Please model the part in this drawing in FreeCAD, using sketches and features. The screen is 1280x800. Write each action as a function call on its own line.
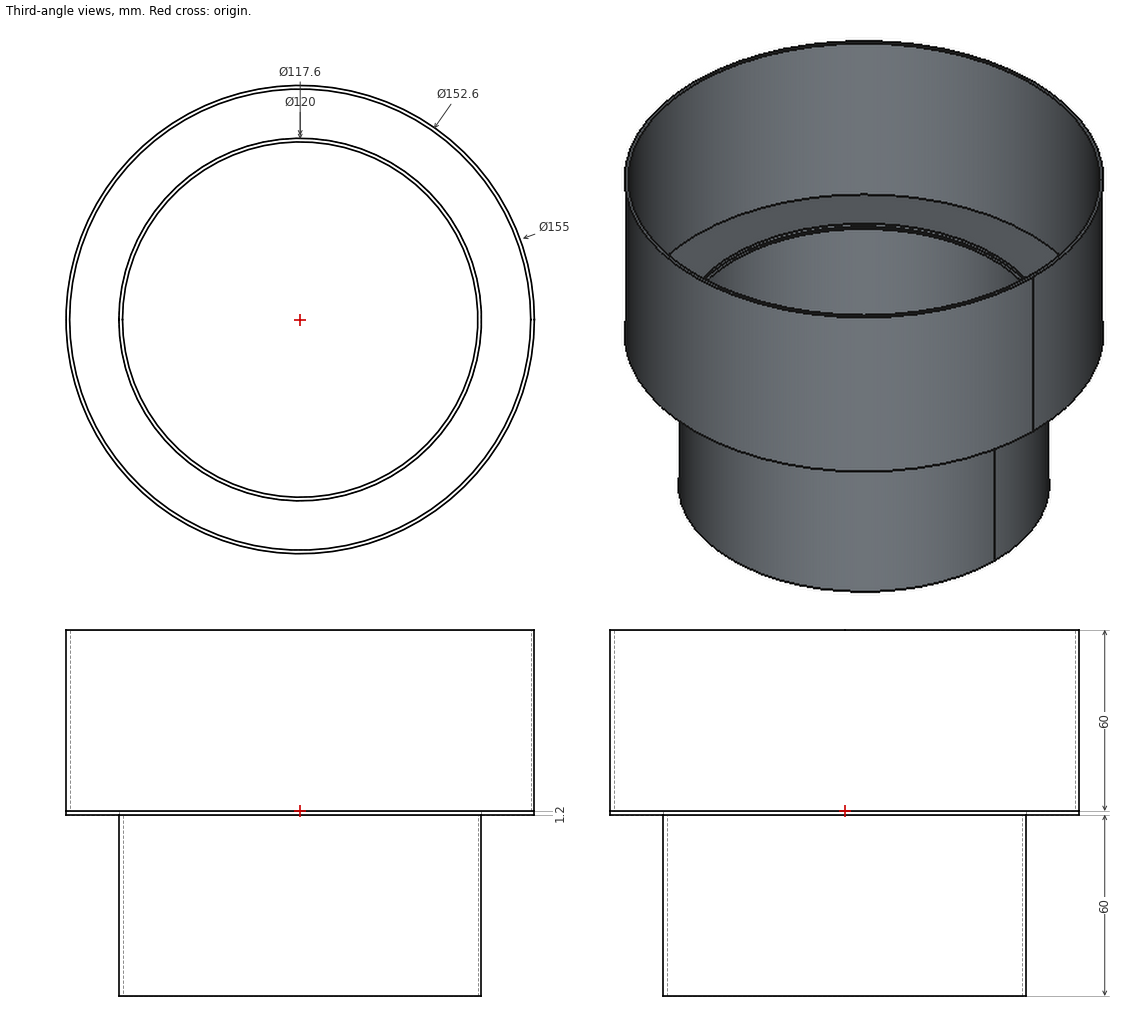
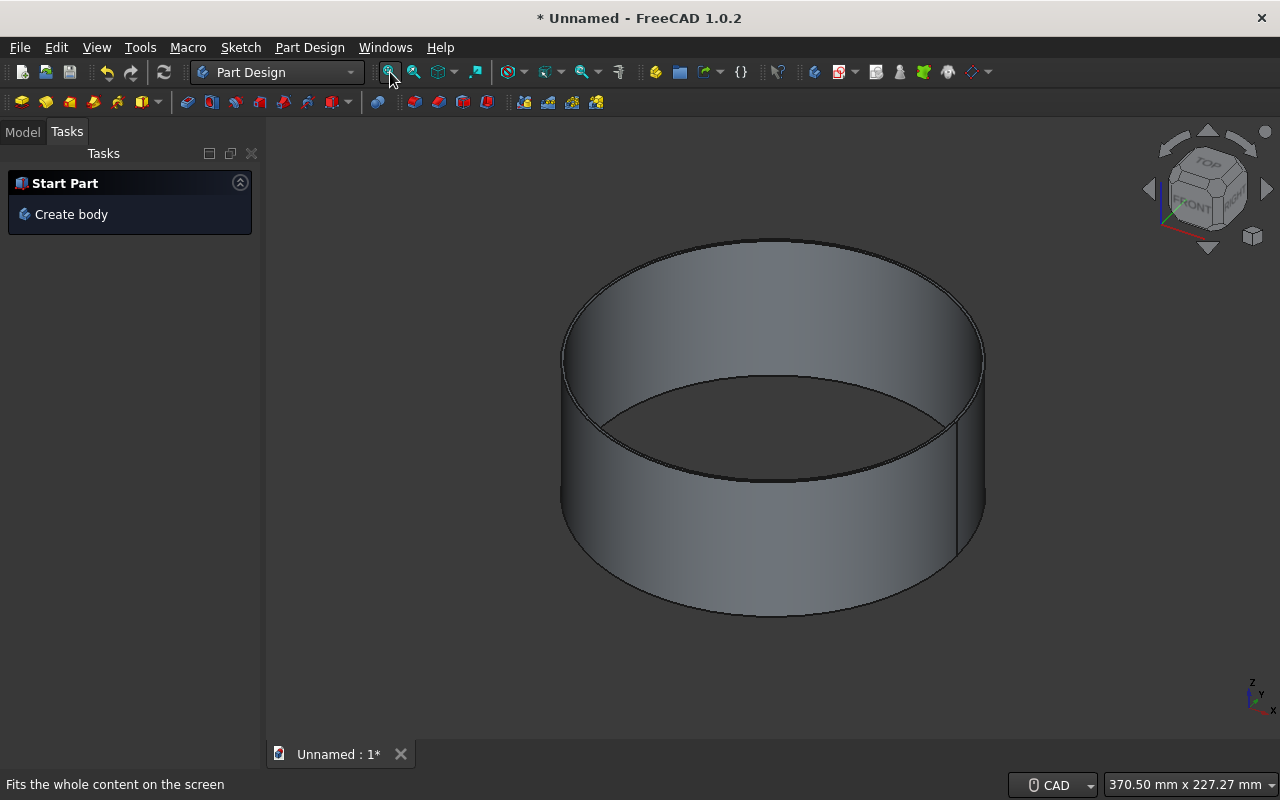
click(23, 131)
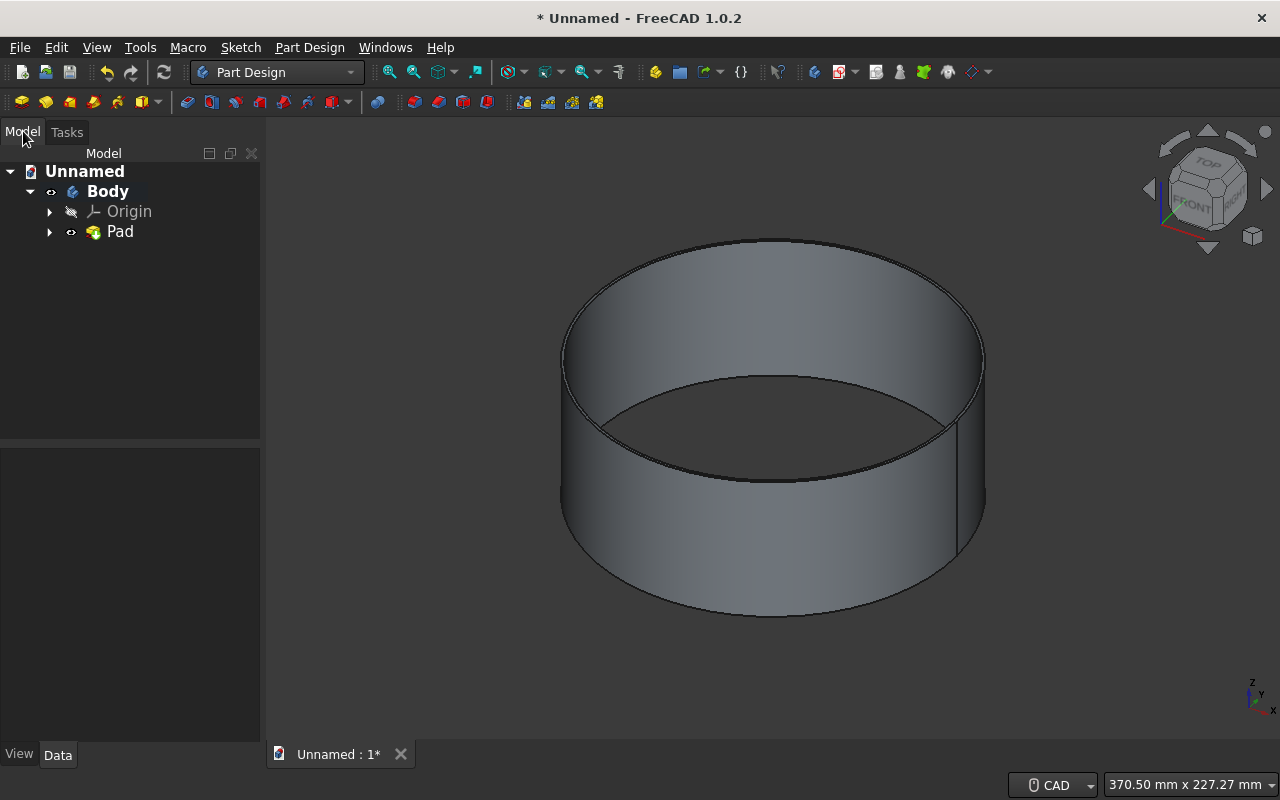
click(50, 212)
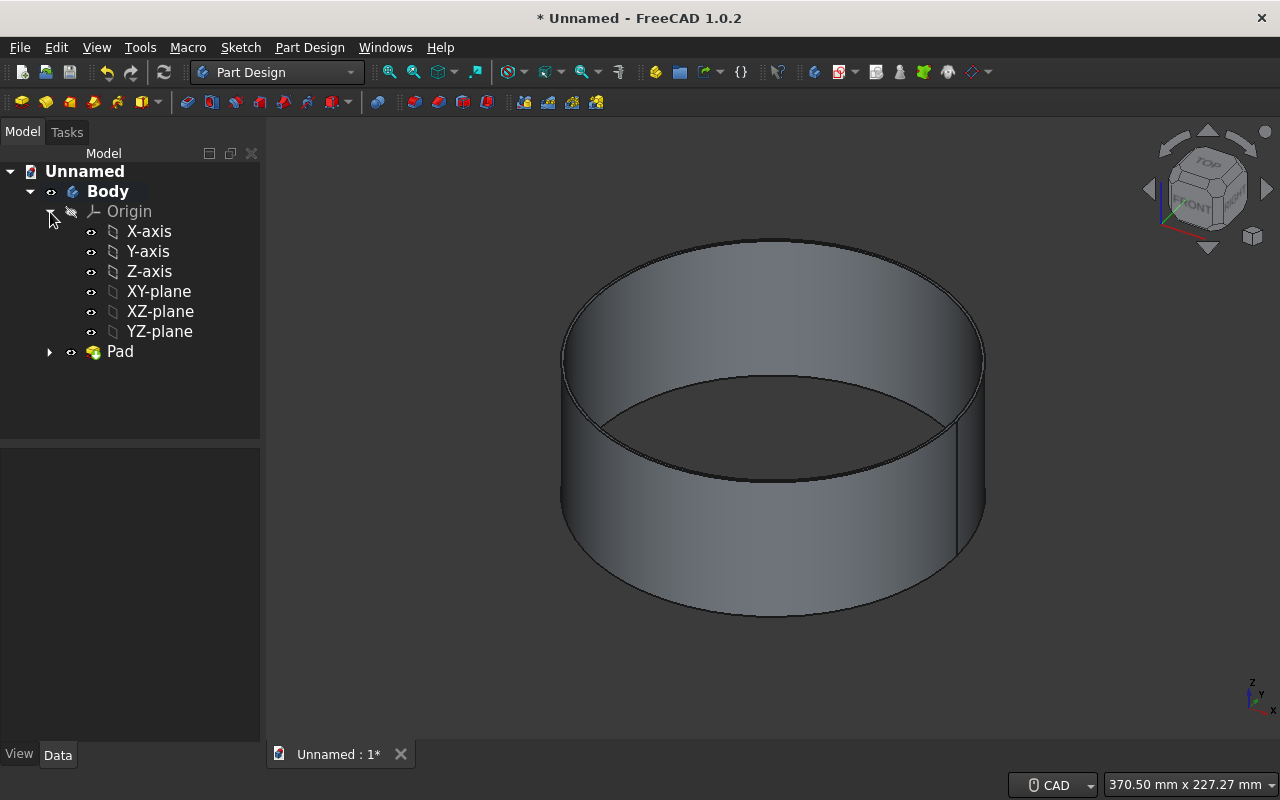
click(136, 292)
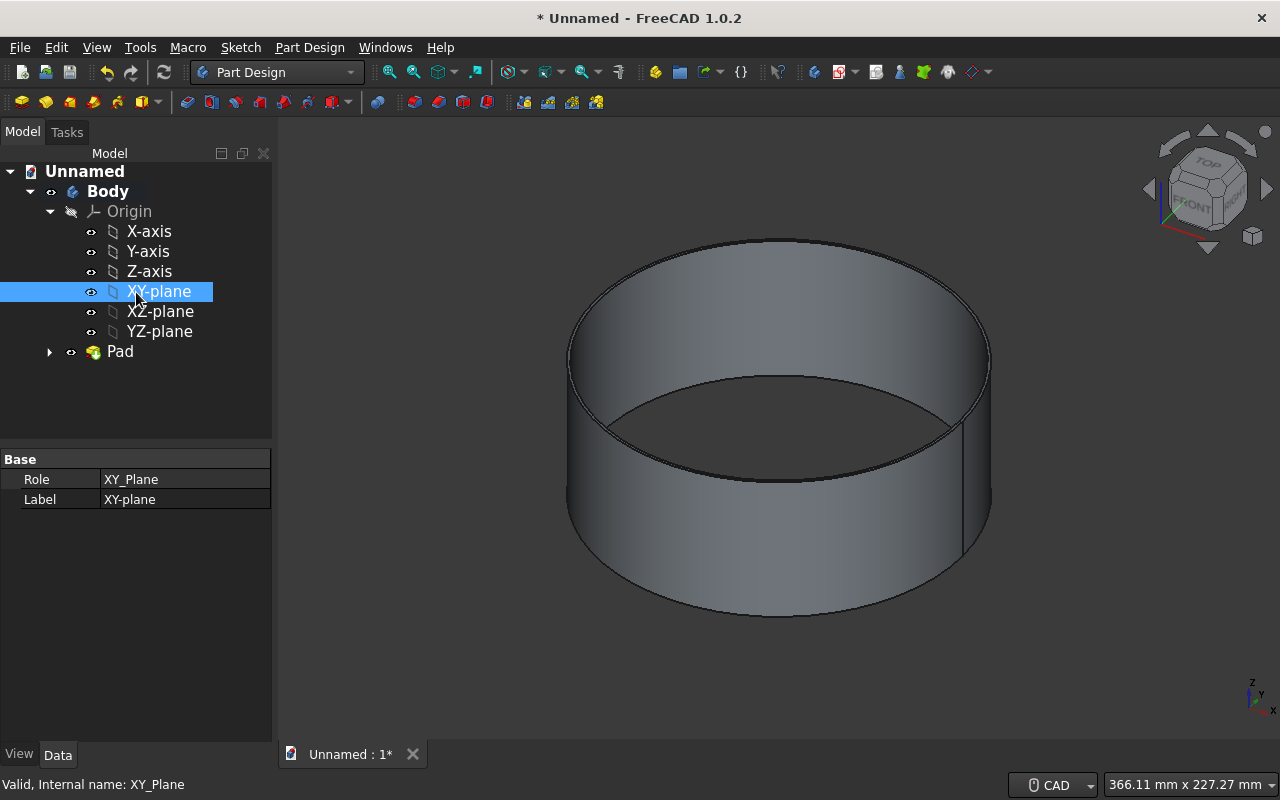
click(972, 72)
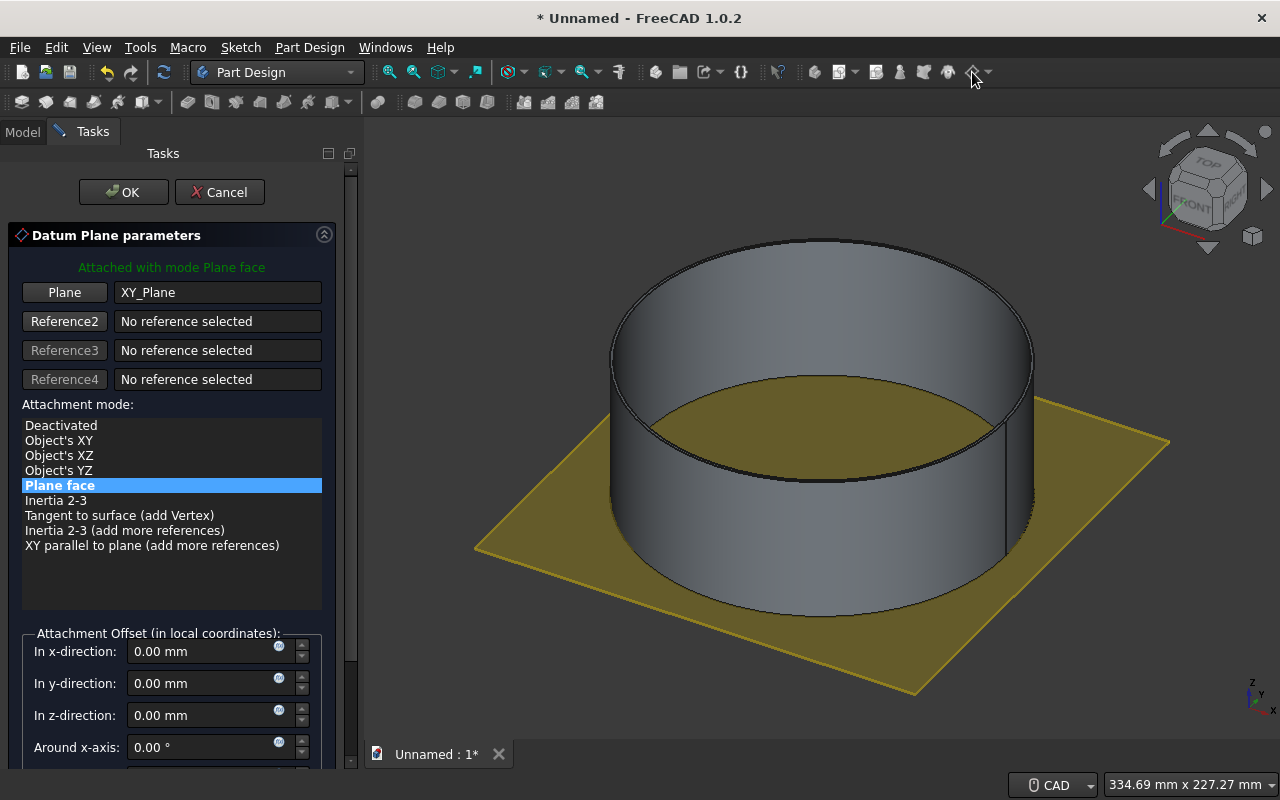
triple_click(210, 715)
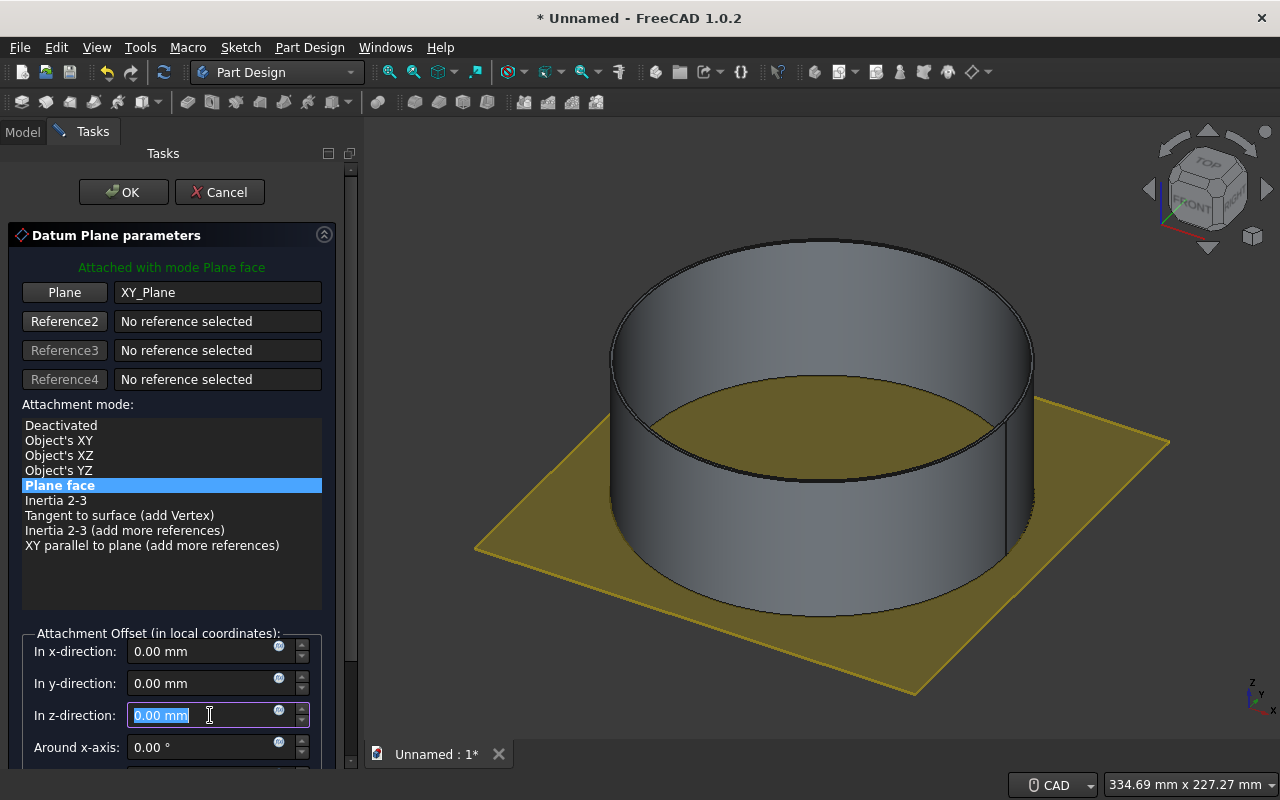
text(-1.2)
key(Tab)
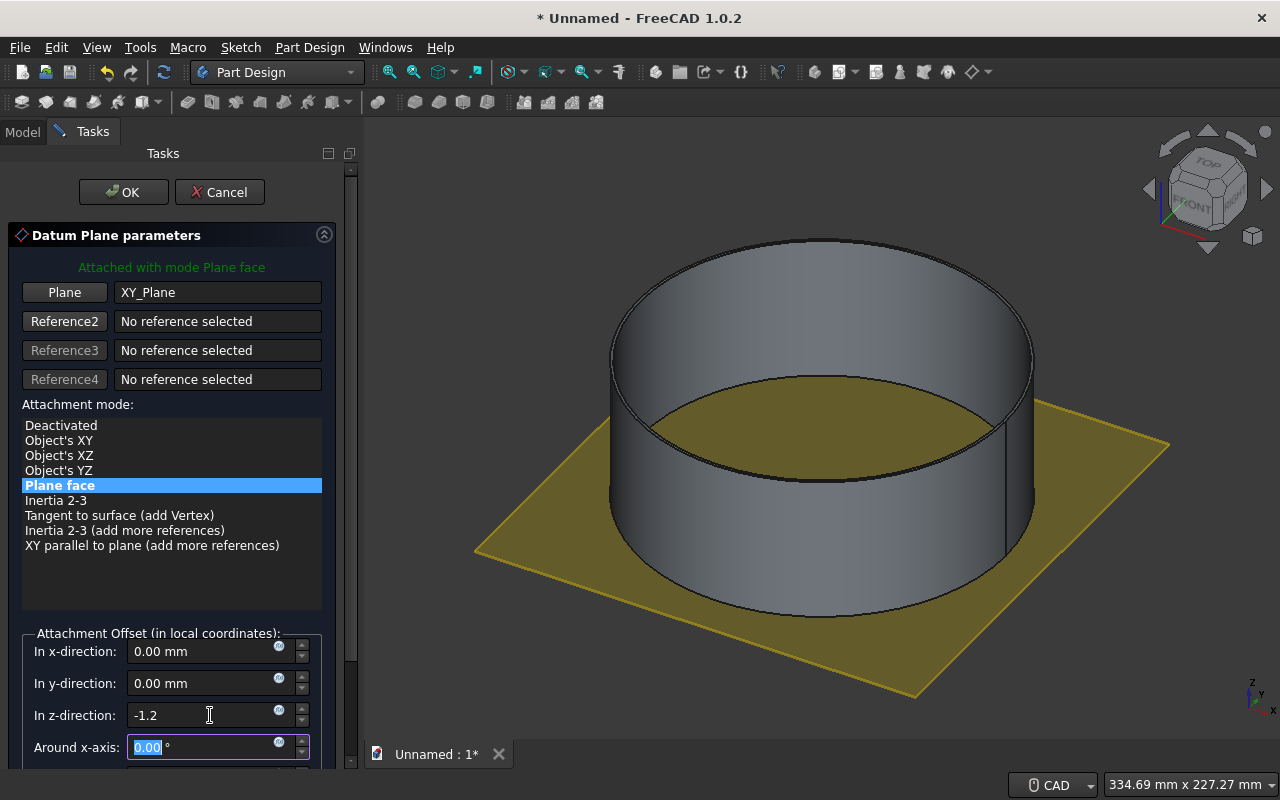
click(124, 192)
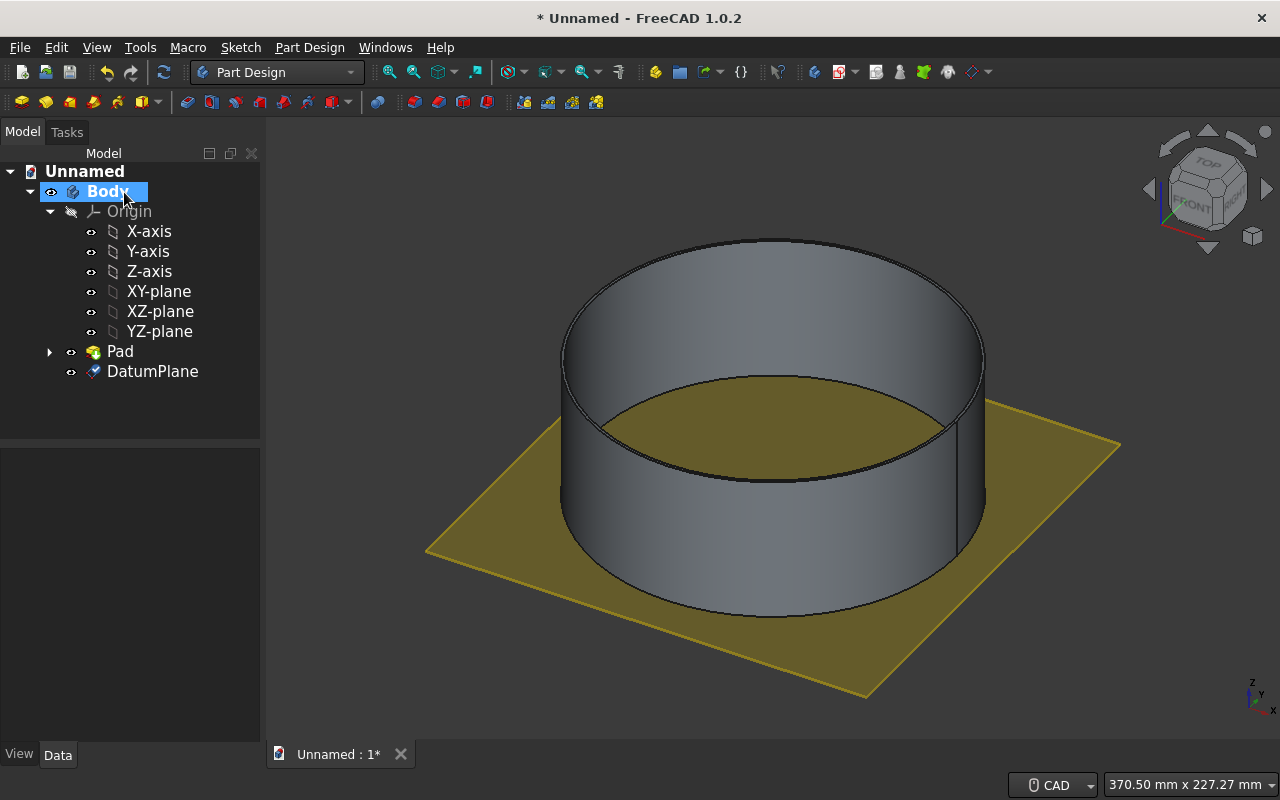
click(116, 372)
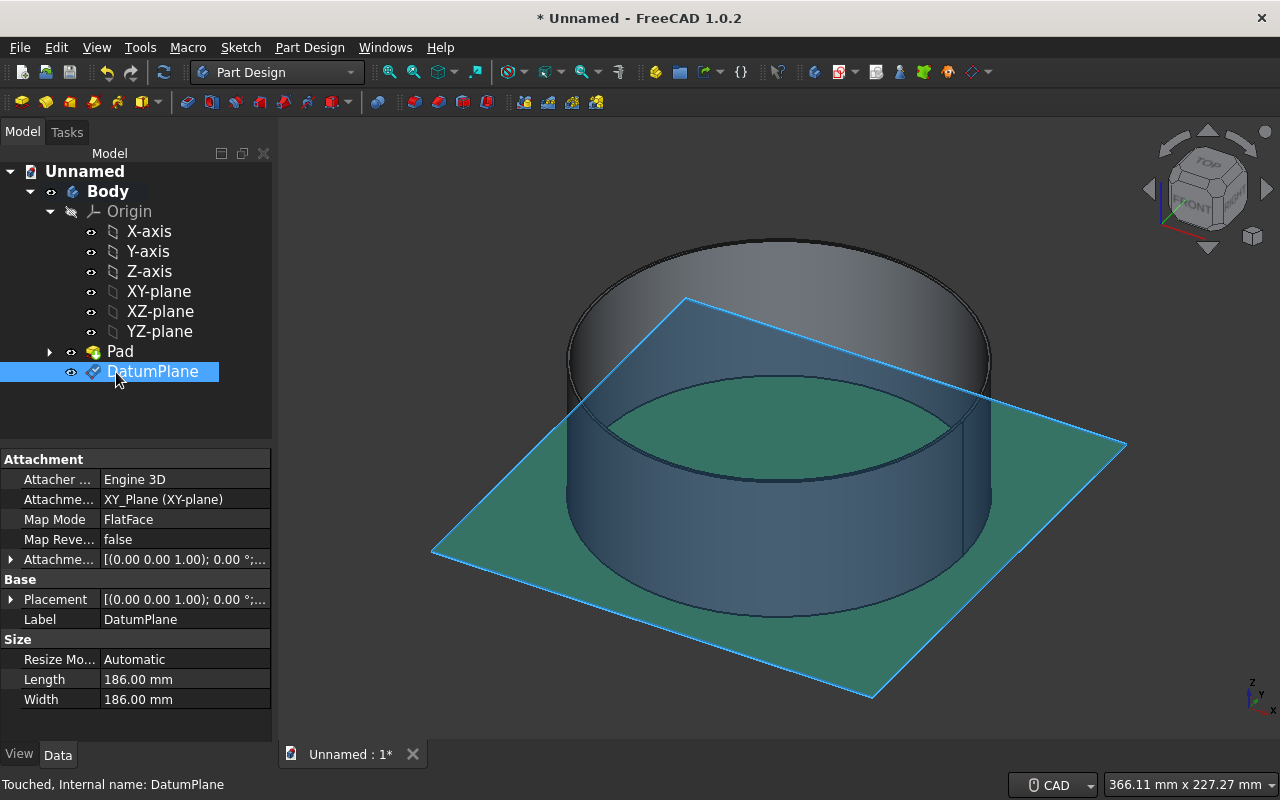
click(840, 72)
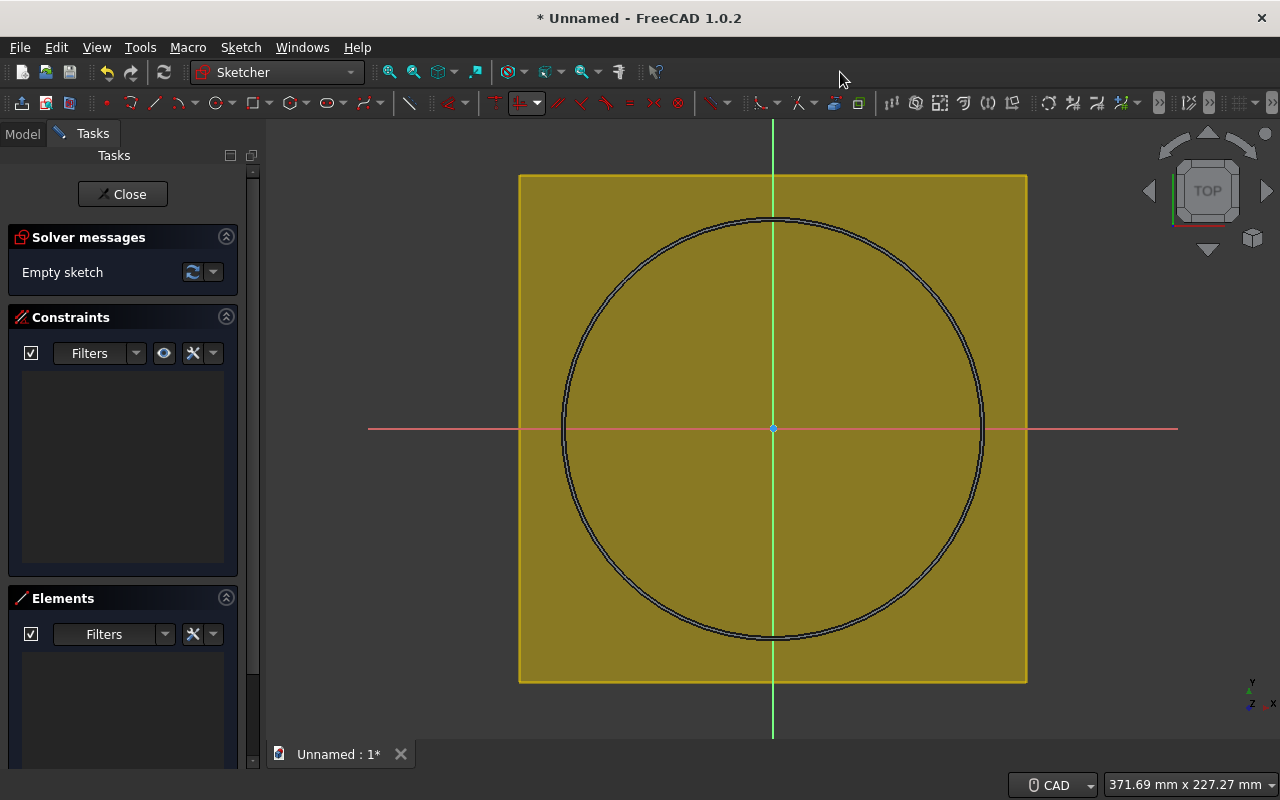
click(70, 104)